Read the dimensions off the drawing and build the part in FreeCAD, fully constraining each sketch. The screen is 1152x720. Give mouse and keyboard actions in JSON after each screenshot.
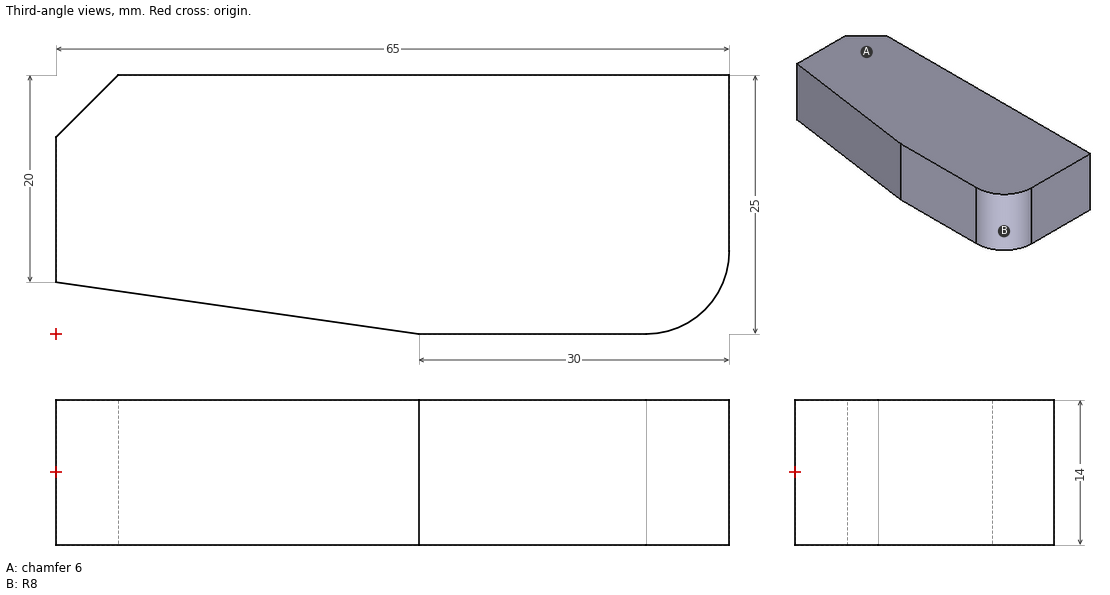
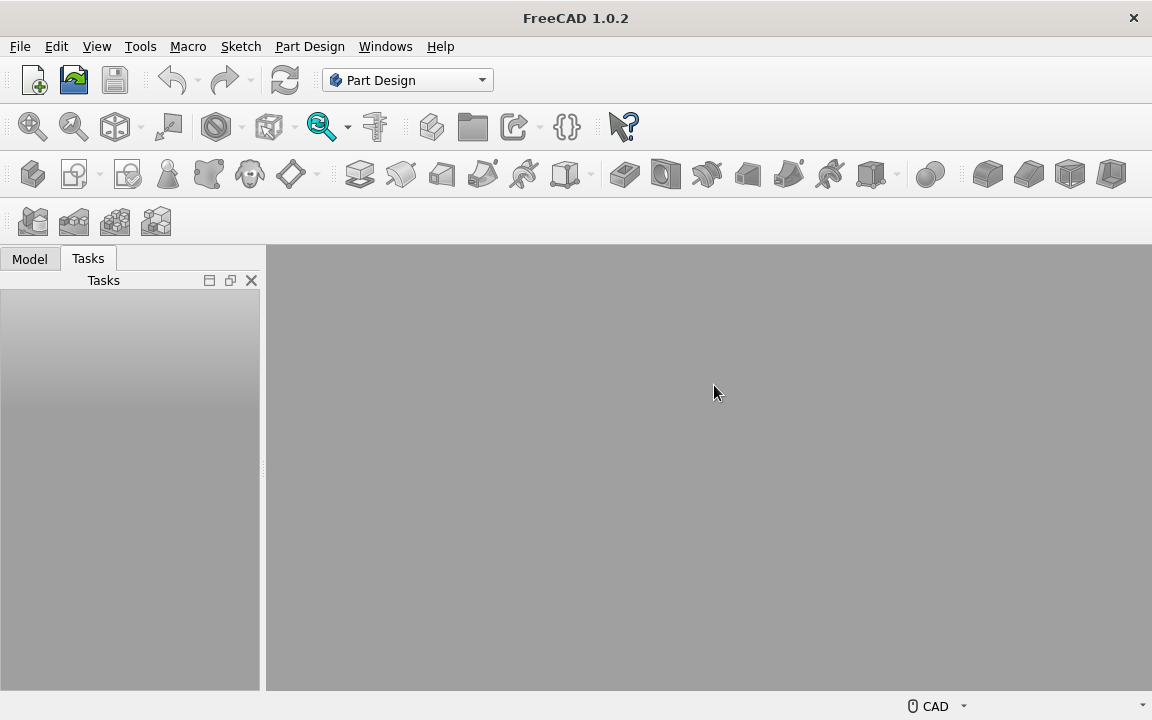
{"action": "left_click", "coordinate": [33, 80]}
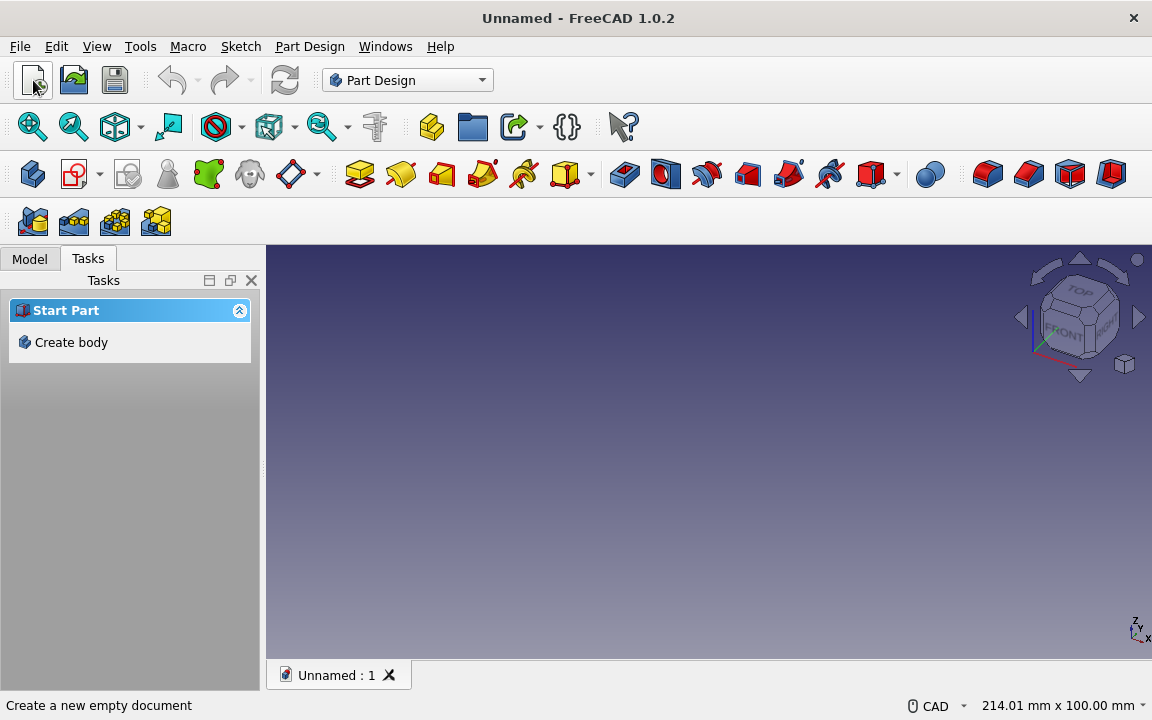
{"action": "left_click", "coordinate": [74, 174]}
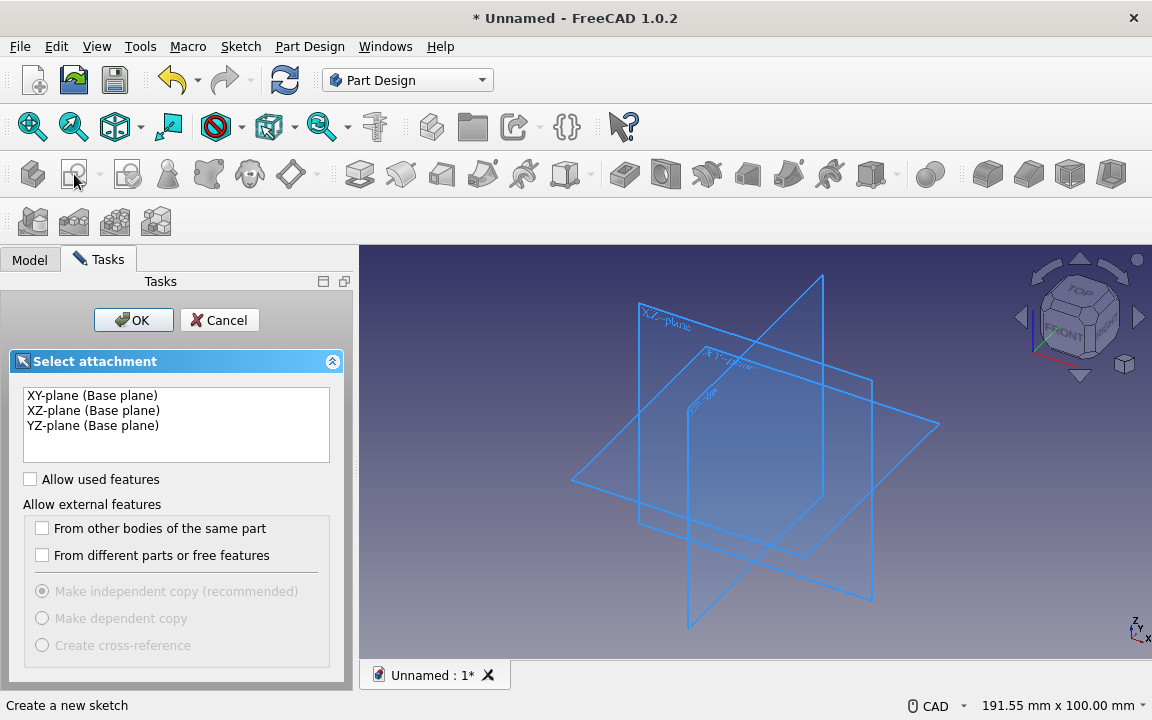
{"action": "left_click", "coordinate": [84, 396]}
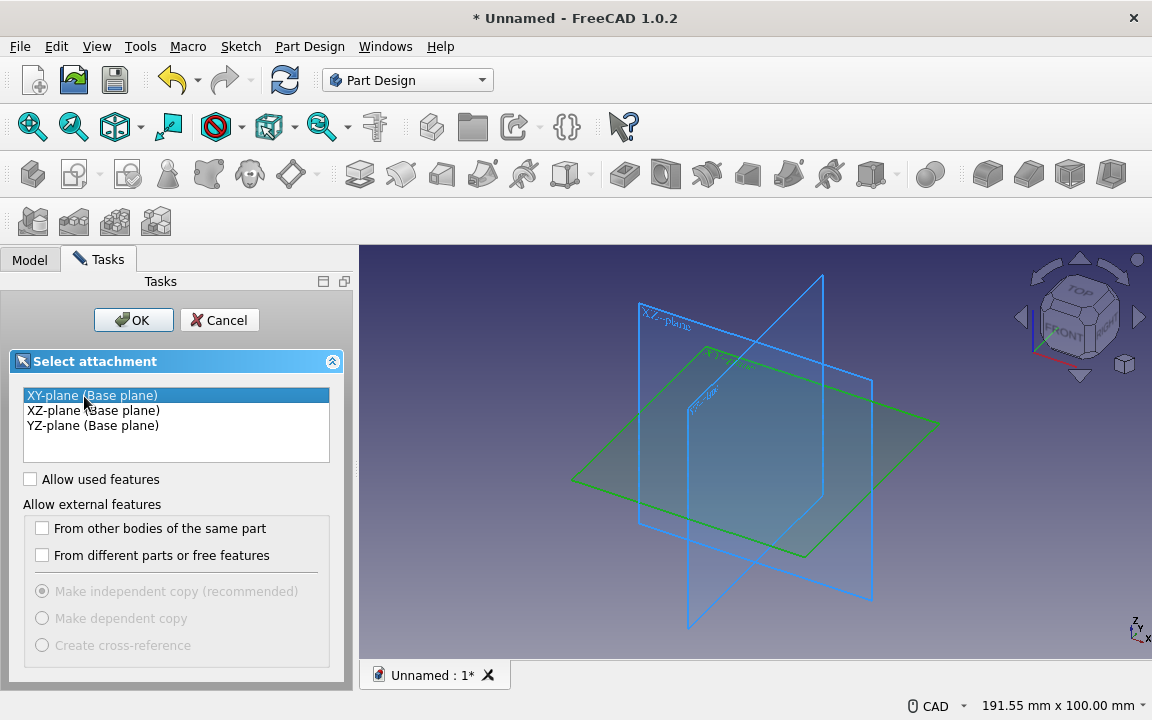
{"action": "left_click", "coordinate": [134, 320]}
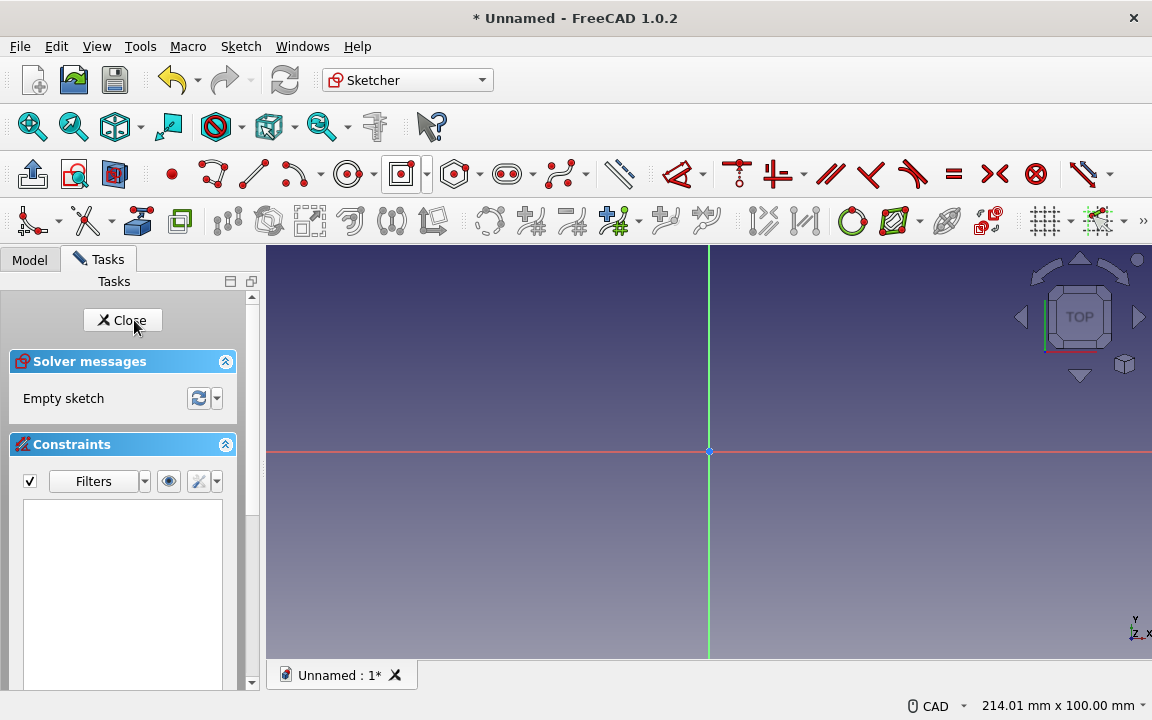
{"action": "scroll", "coordinate": [640, 452], "scroll_direction": "down", "scroll_amount": 5}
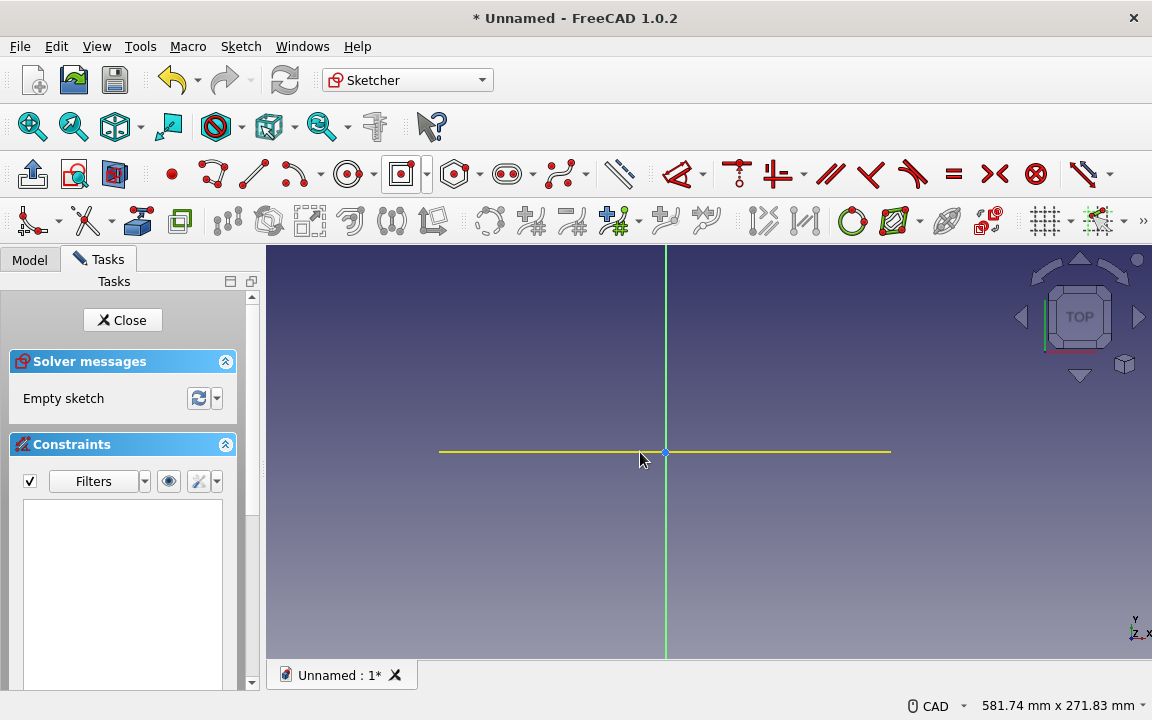
{"action": "scroll", "coordinate": [734, 429], "scroll_direction": "up", "scroll_amount": 8}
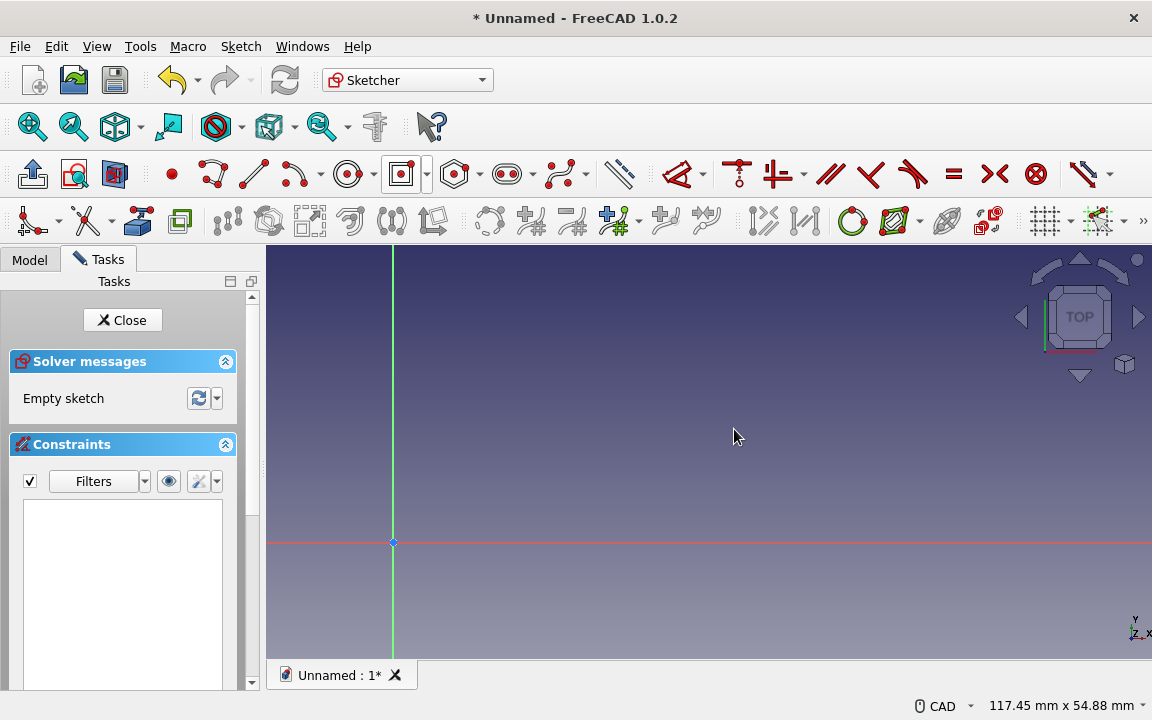
{"action": "left_click", "coordinate": [213, 174]}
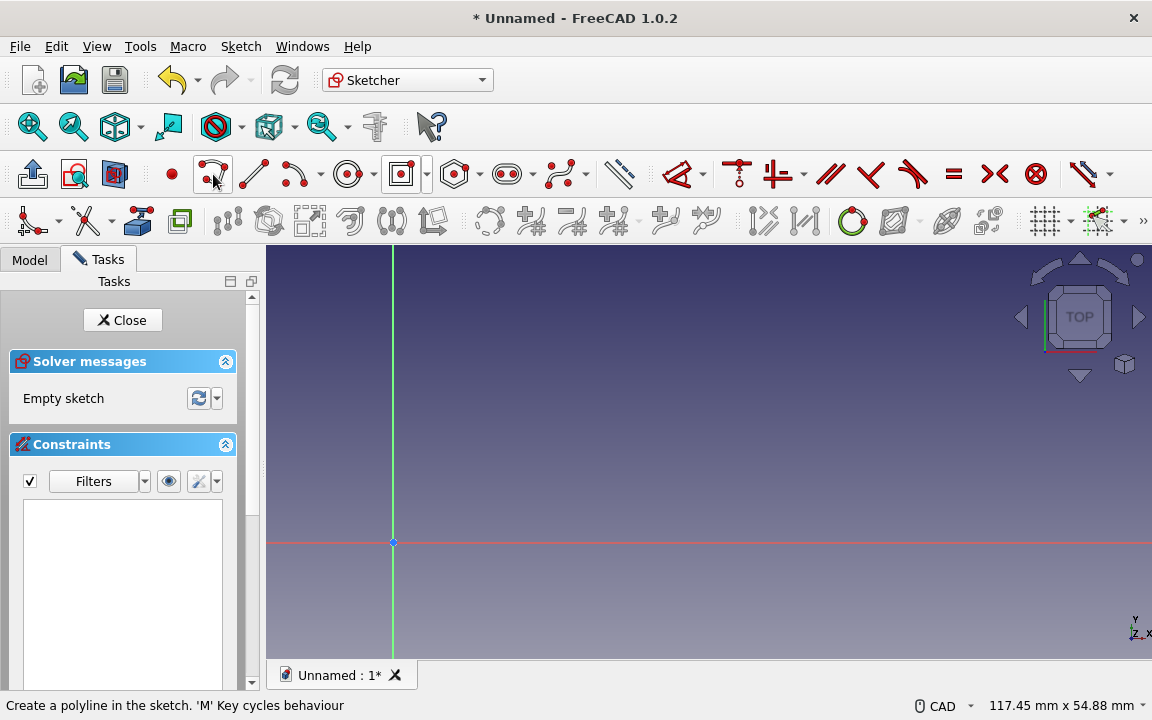
{"action": "left_click", "coordinate": [393, 505]}
{"action": "left_click", "coordinate": [657, 543]}
{"action": "left_click", "coordinate": [884, 534]}
{"action": "left_click", "coordinate": [884, 354]}
{"action": "left_click", "coordinate": [402, 354]}
{"action": "left_click", "coordinate": [393, 506]}
{"action": "key", "text": "Escape"}
{"action": "key", "text": "Escape"}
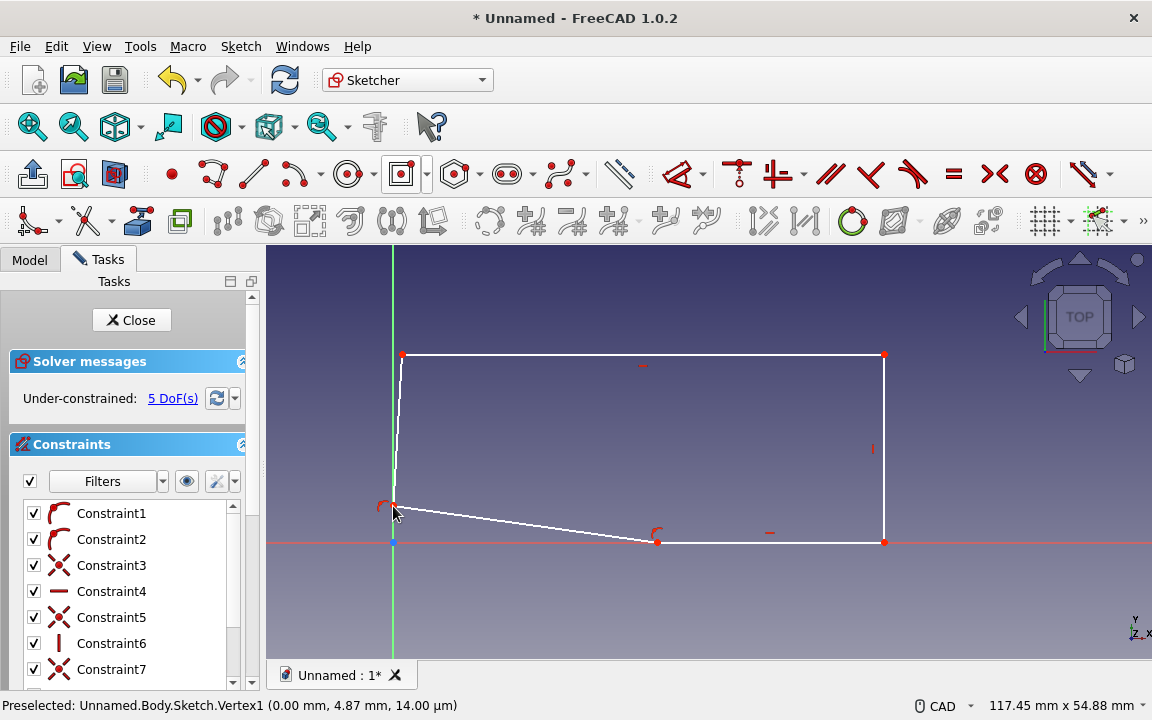
{"action": "left_click", "coordinate": [396, 461]}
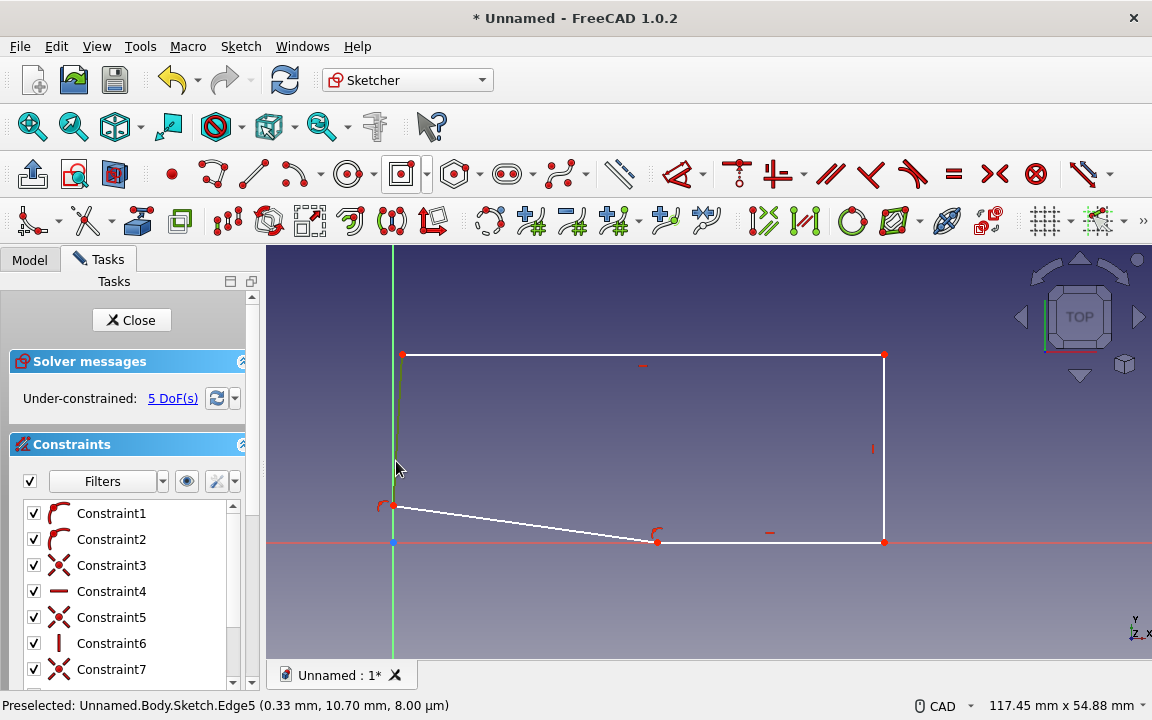
{"action": "key", "text": "v"}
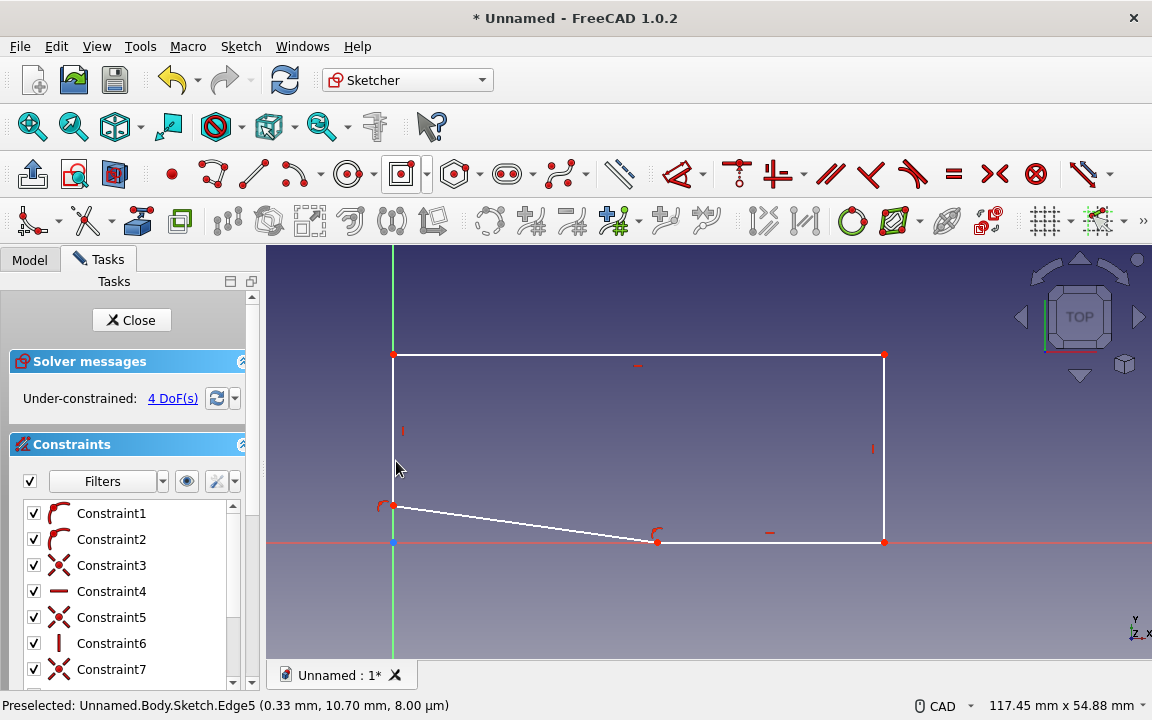
{"action": "left_click", "coordinate": [676, 174]}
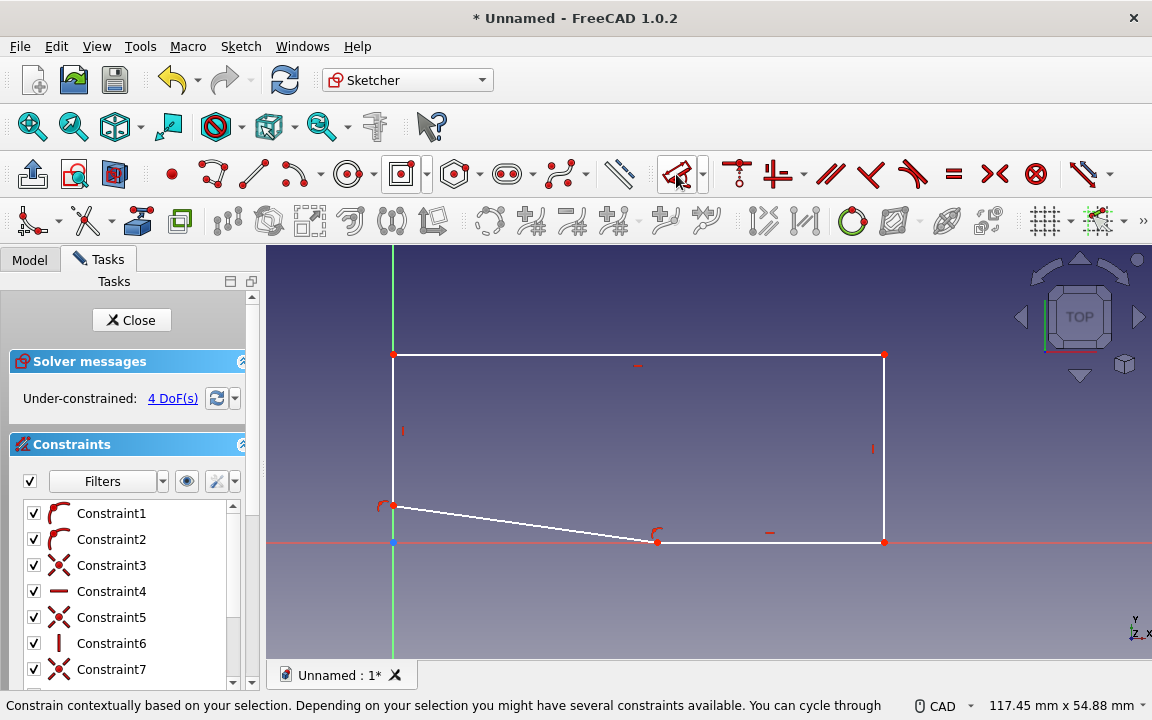
{"action": "left_click", "coordinate": [725, 543]}
{"action": "left_click", "coordinate": [770, 577]}